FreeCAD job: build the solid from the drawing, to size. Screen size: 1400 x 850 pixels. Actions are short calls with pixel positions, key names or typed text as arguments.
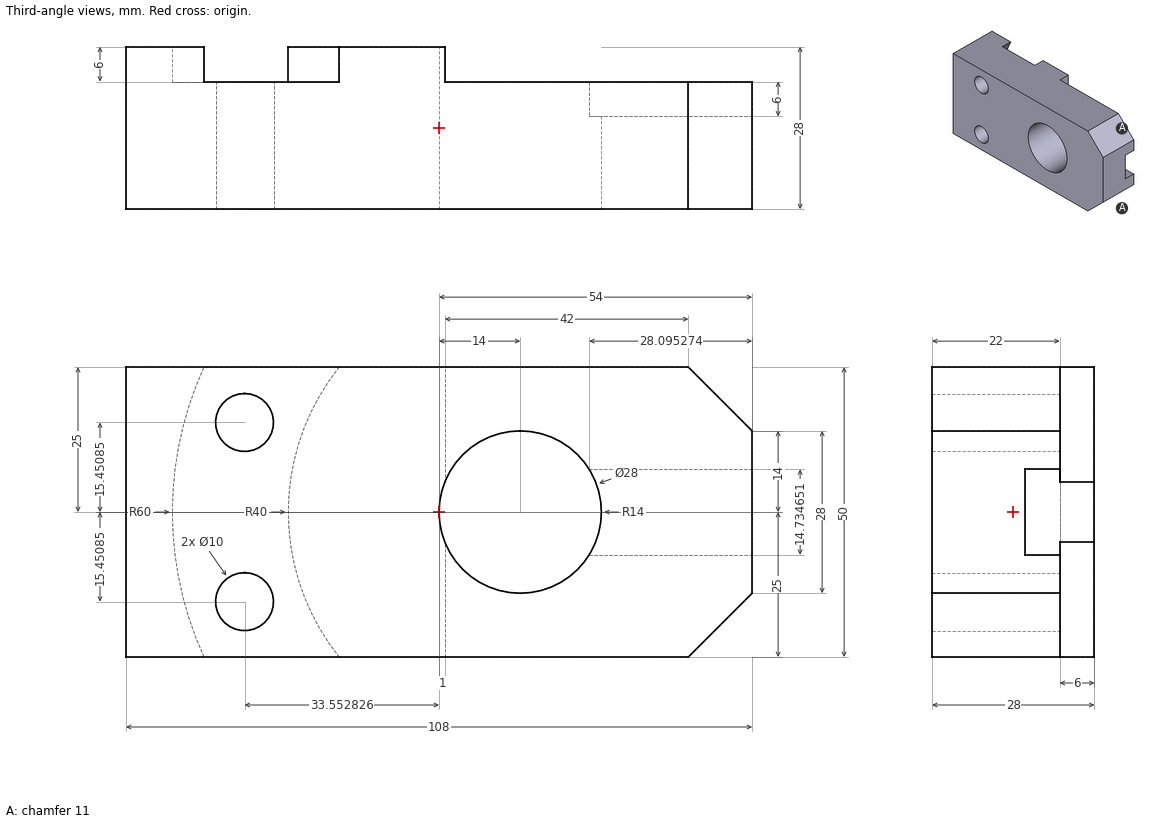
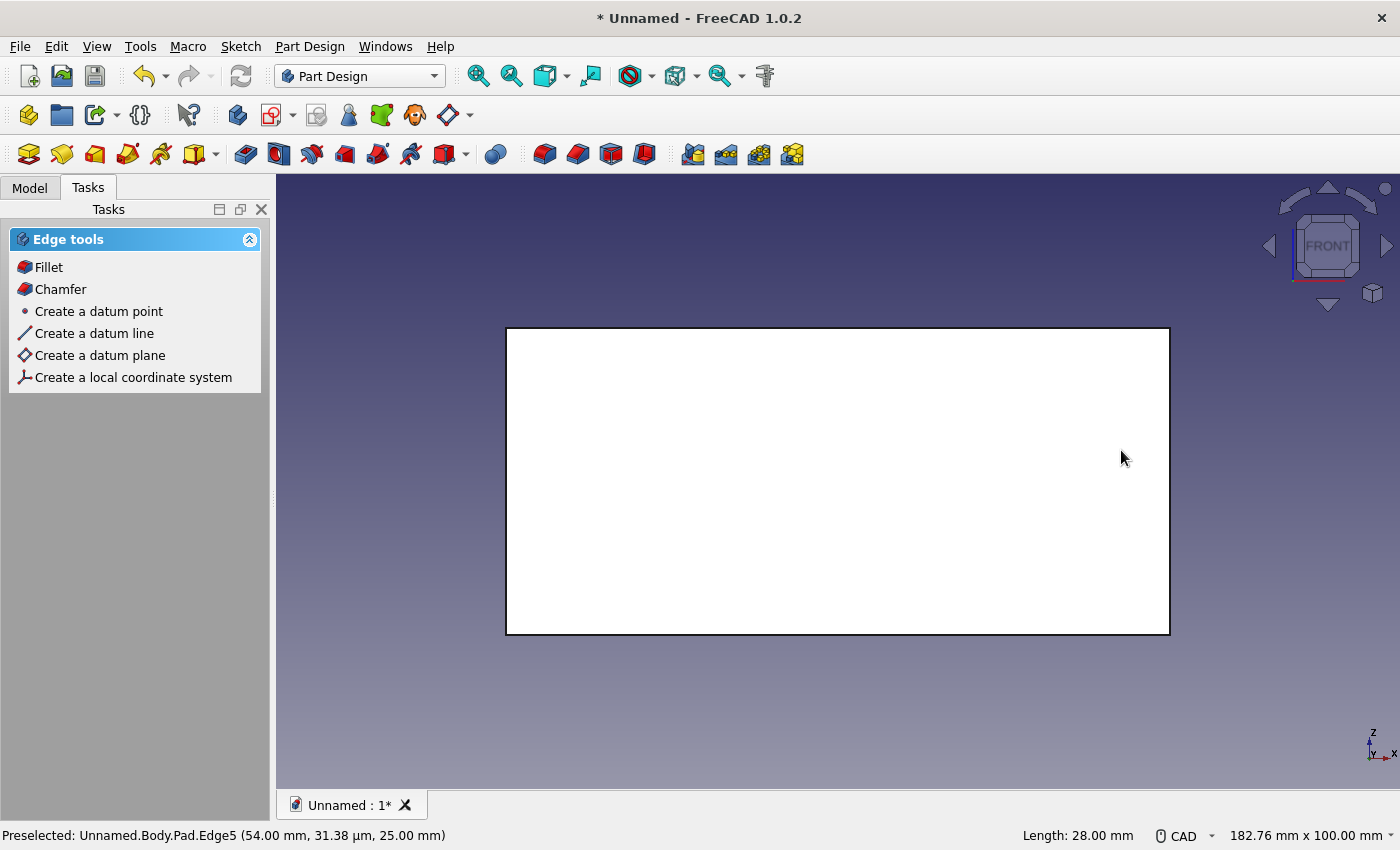
key(3)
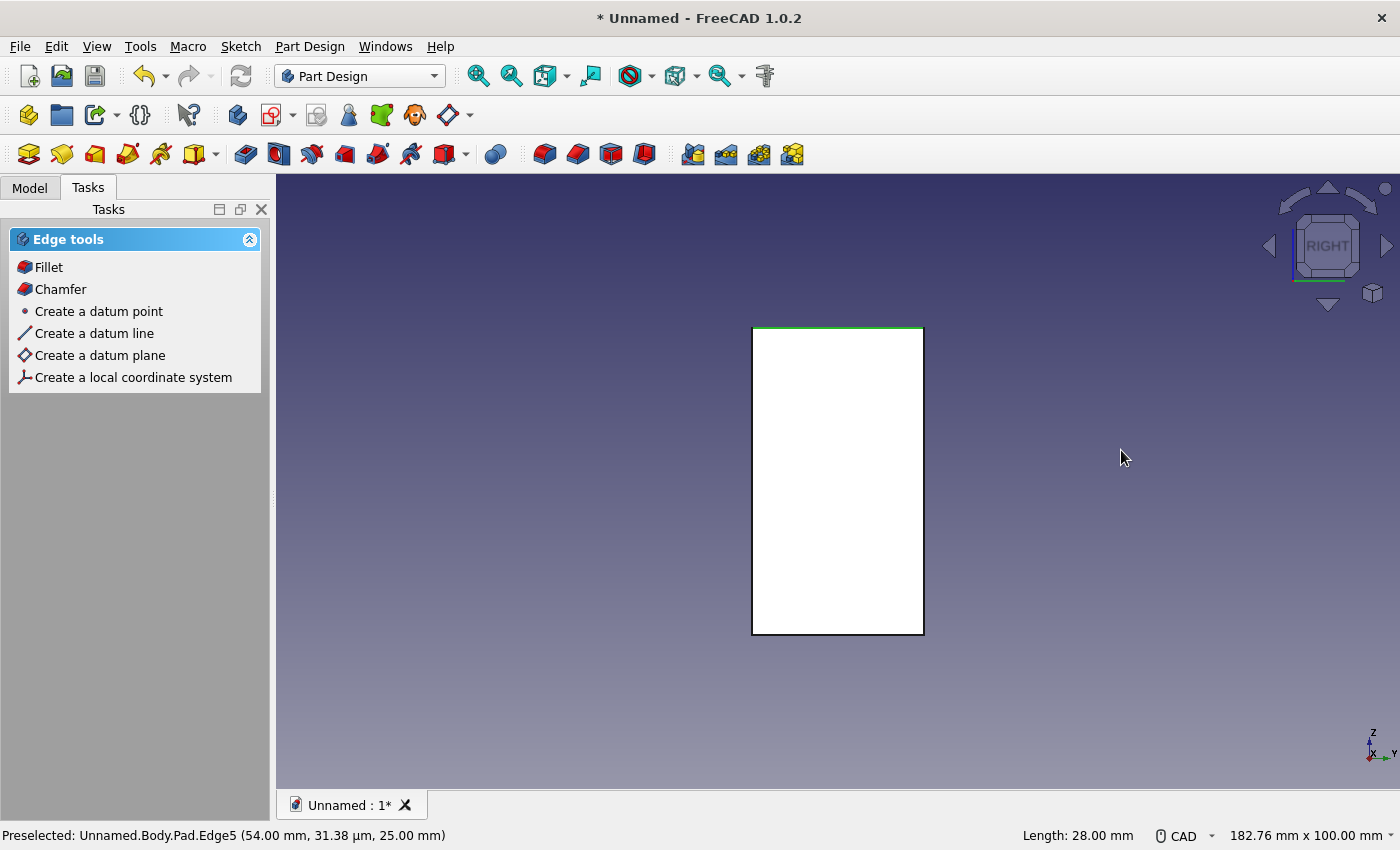
click(838, 634, ctrl)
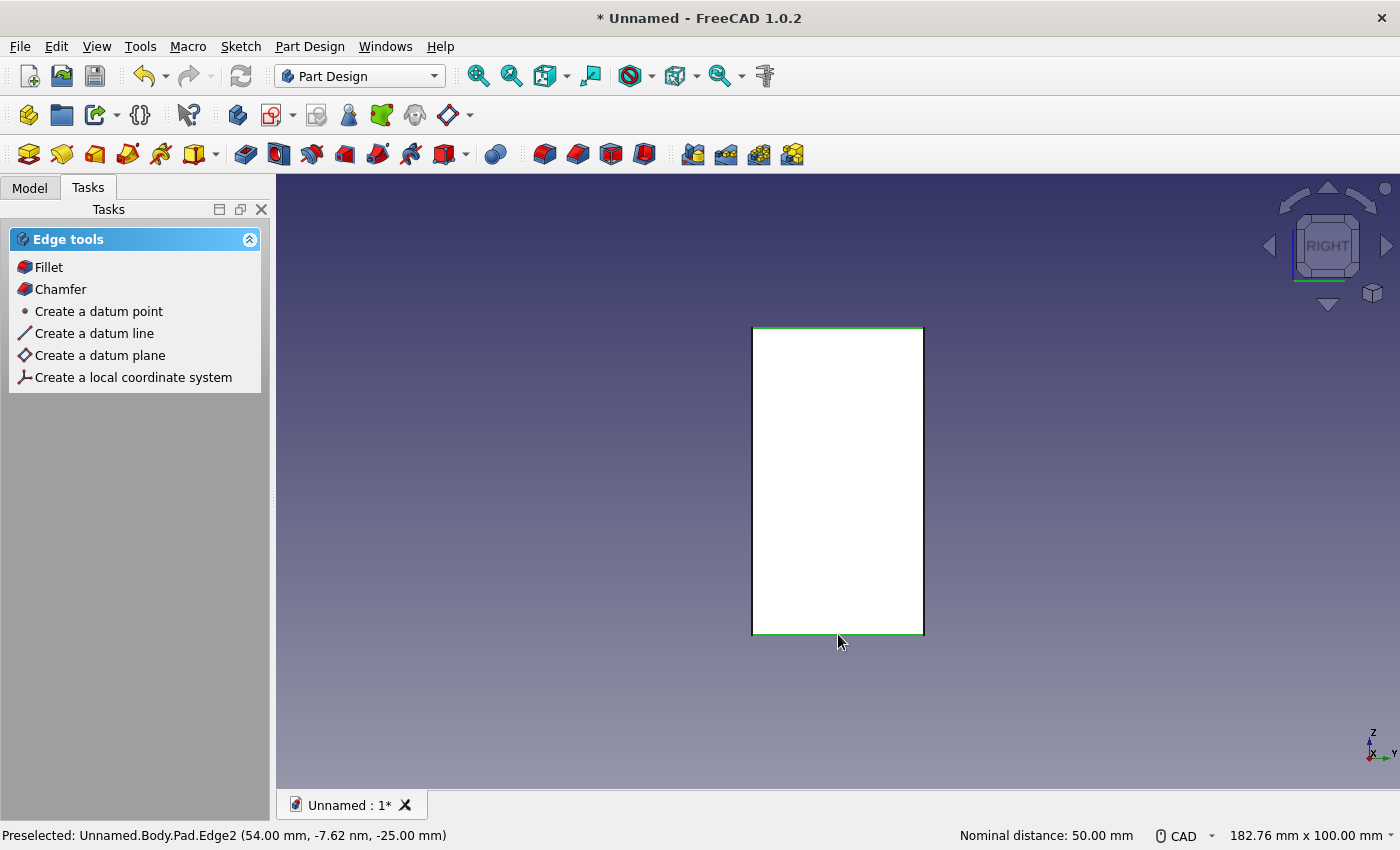
click(578, 154)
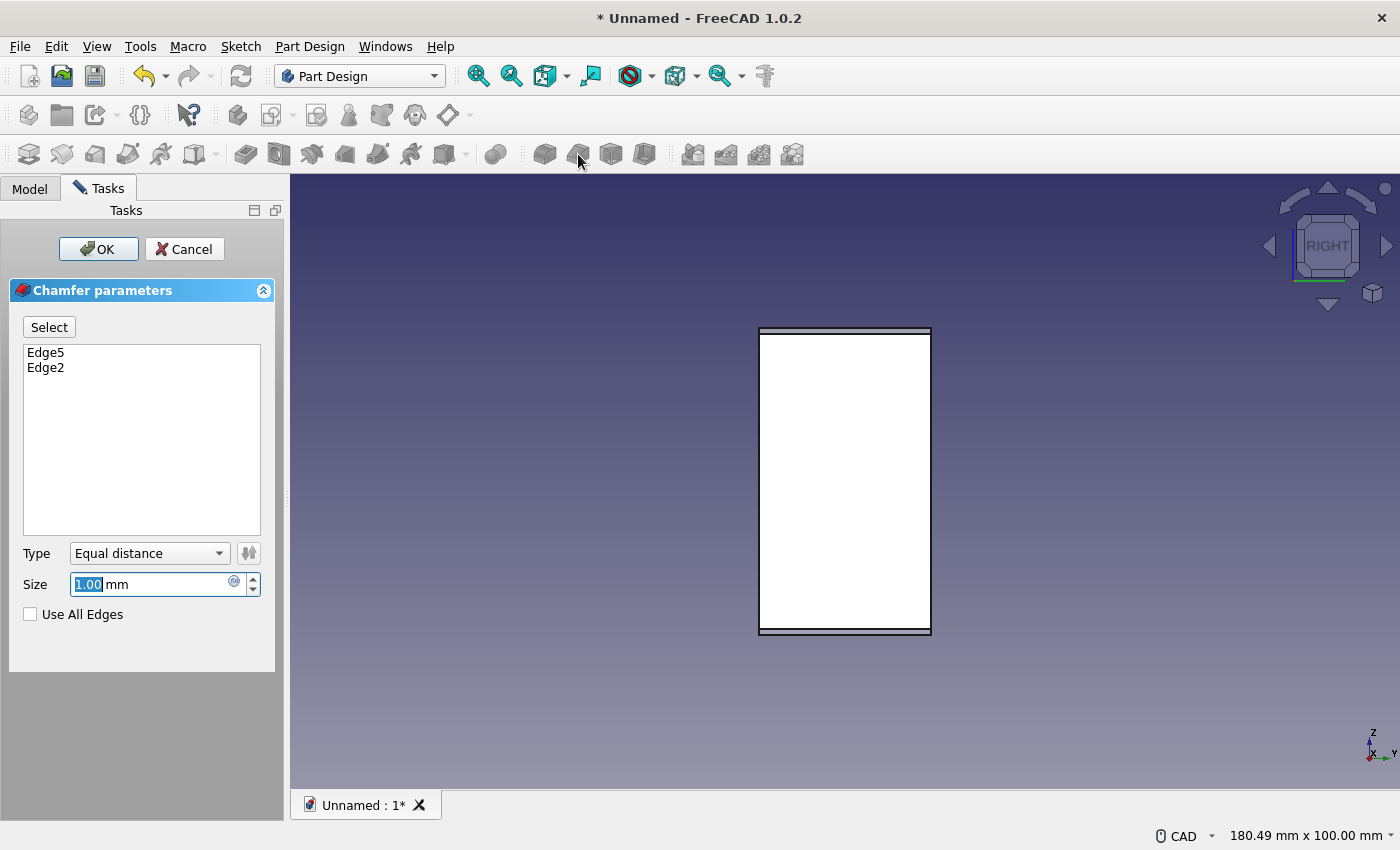
text(11)
key(Tab)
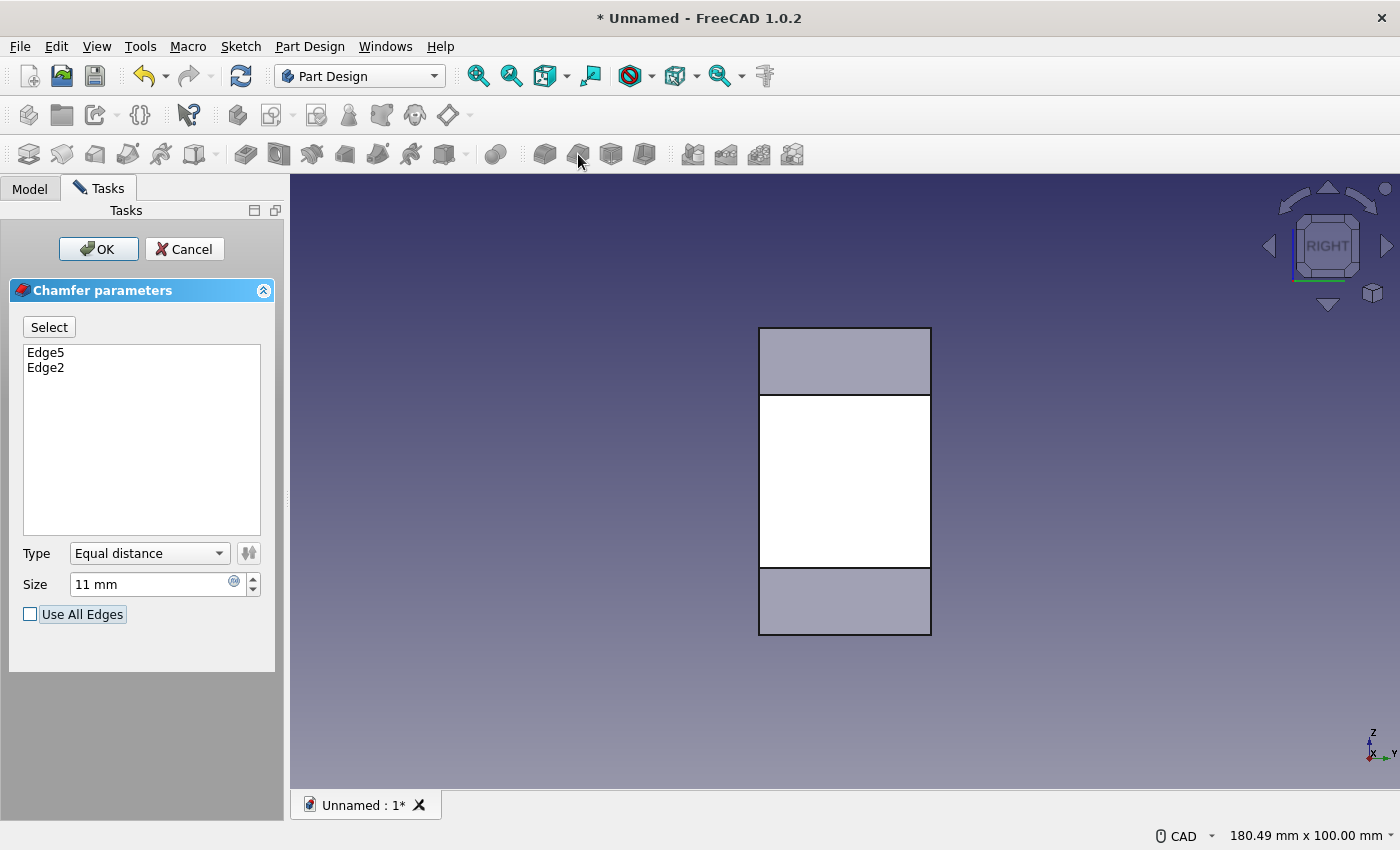
click(99, 249)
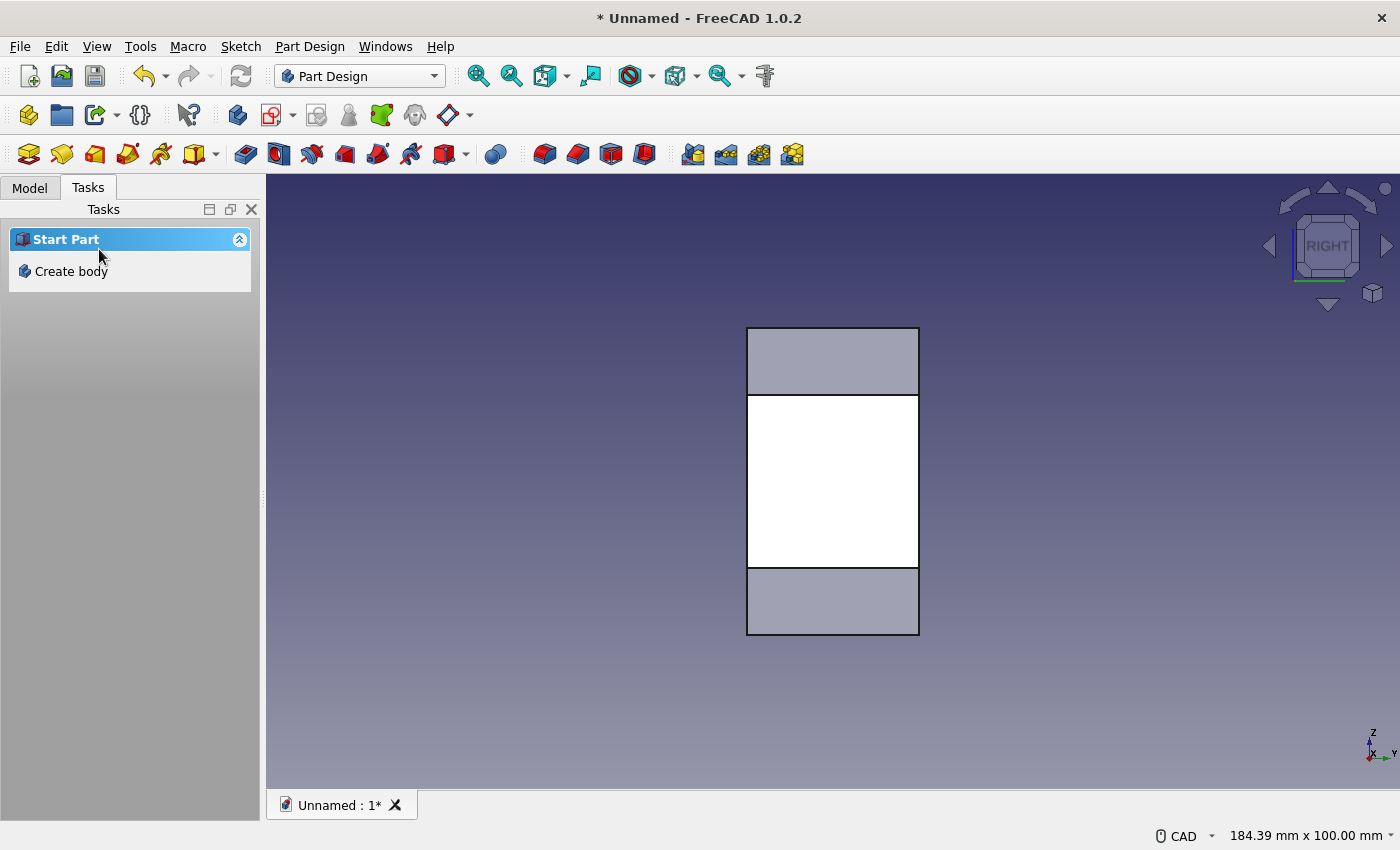
key(4)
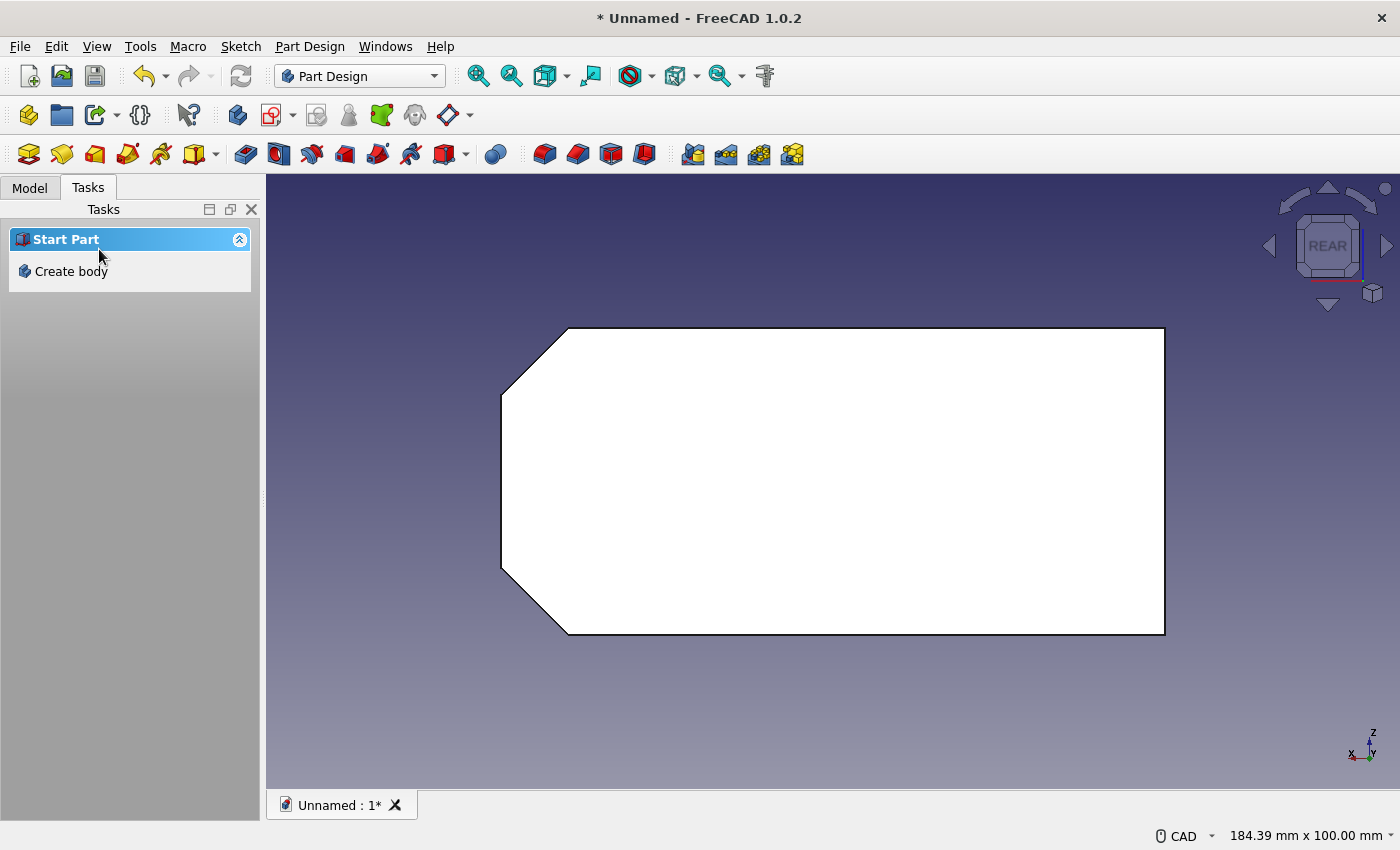
click(738, 480)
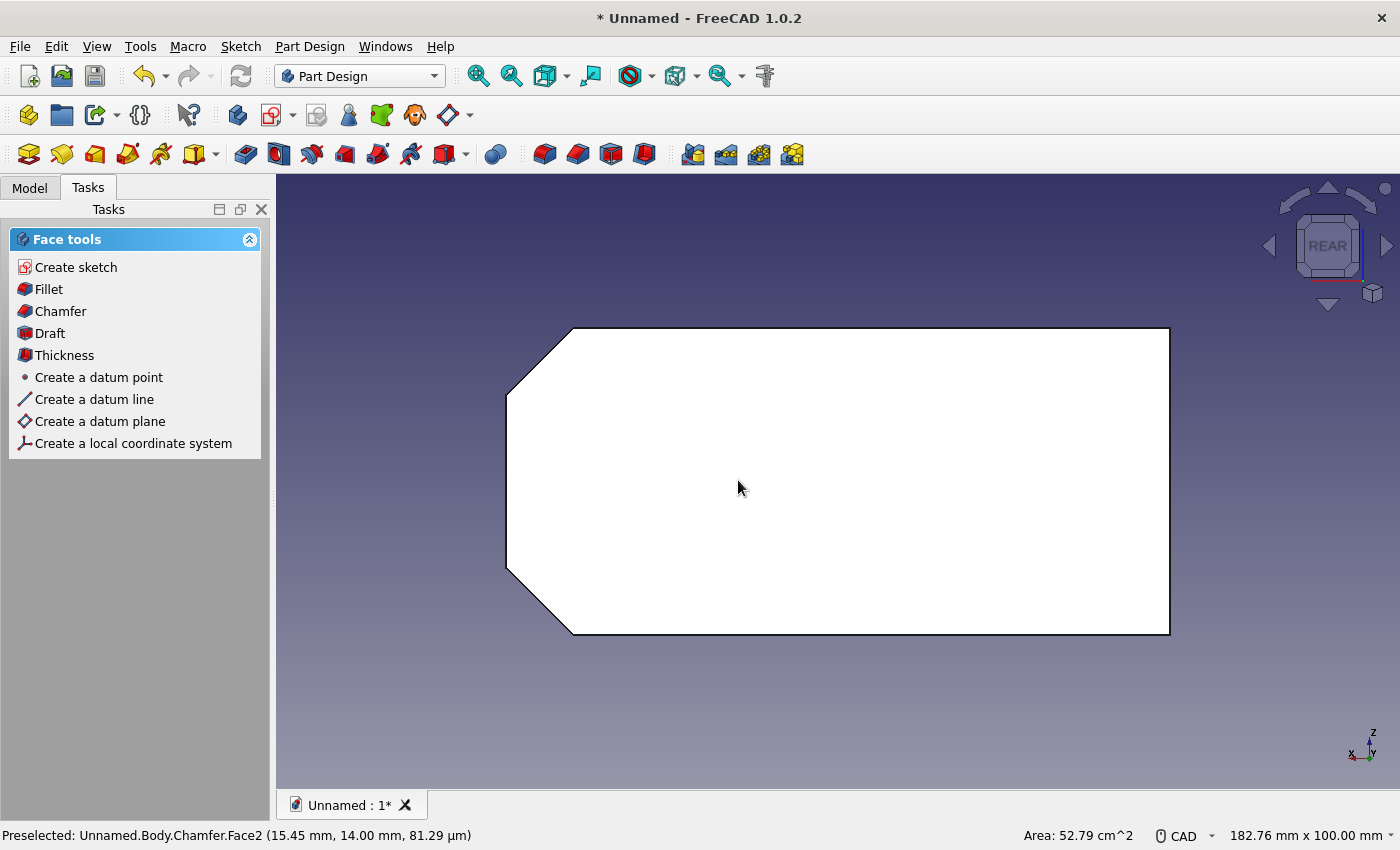
click(270, 116)